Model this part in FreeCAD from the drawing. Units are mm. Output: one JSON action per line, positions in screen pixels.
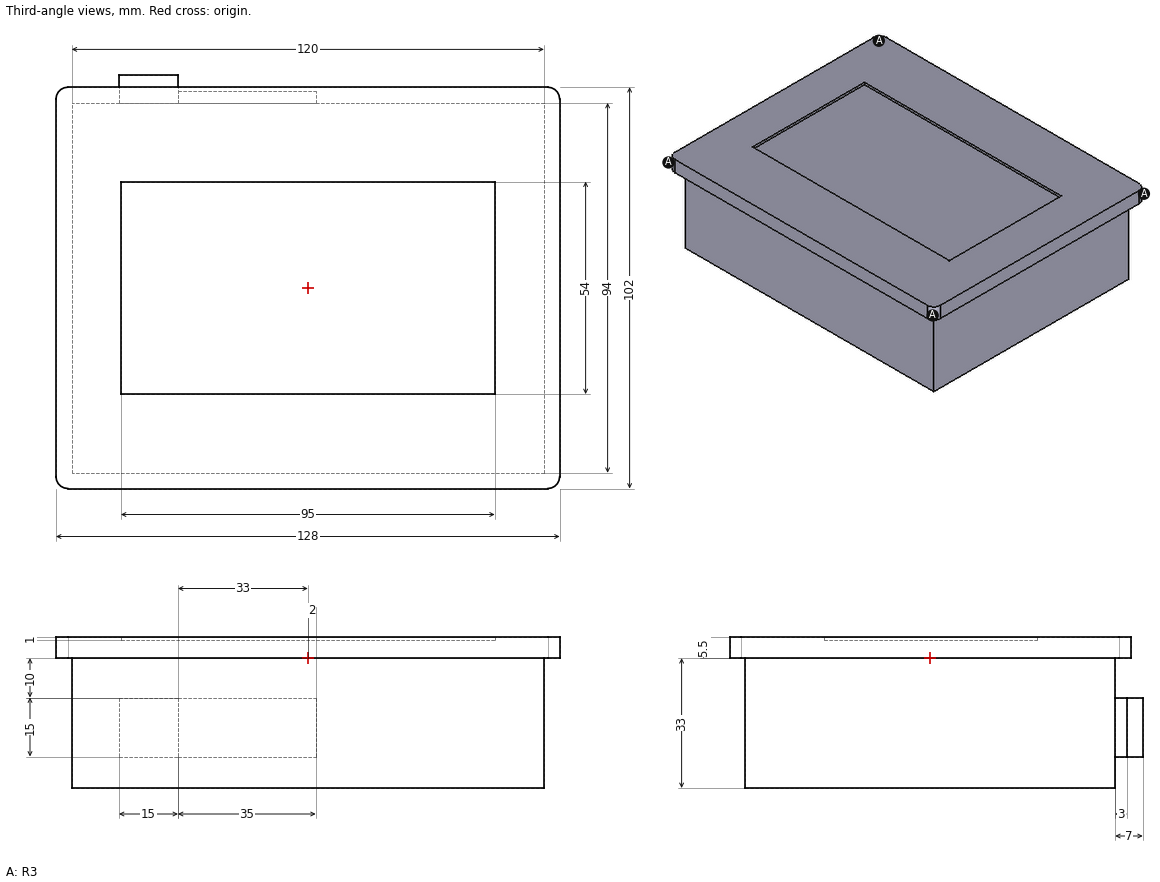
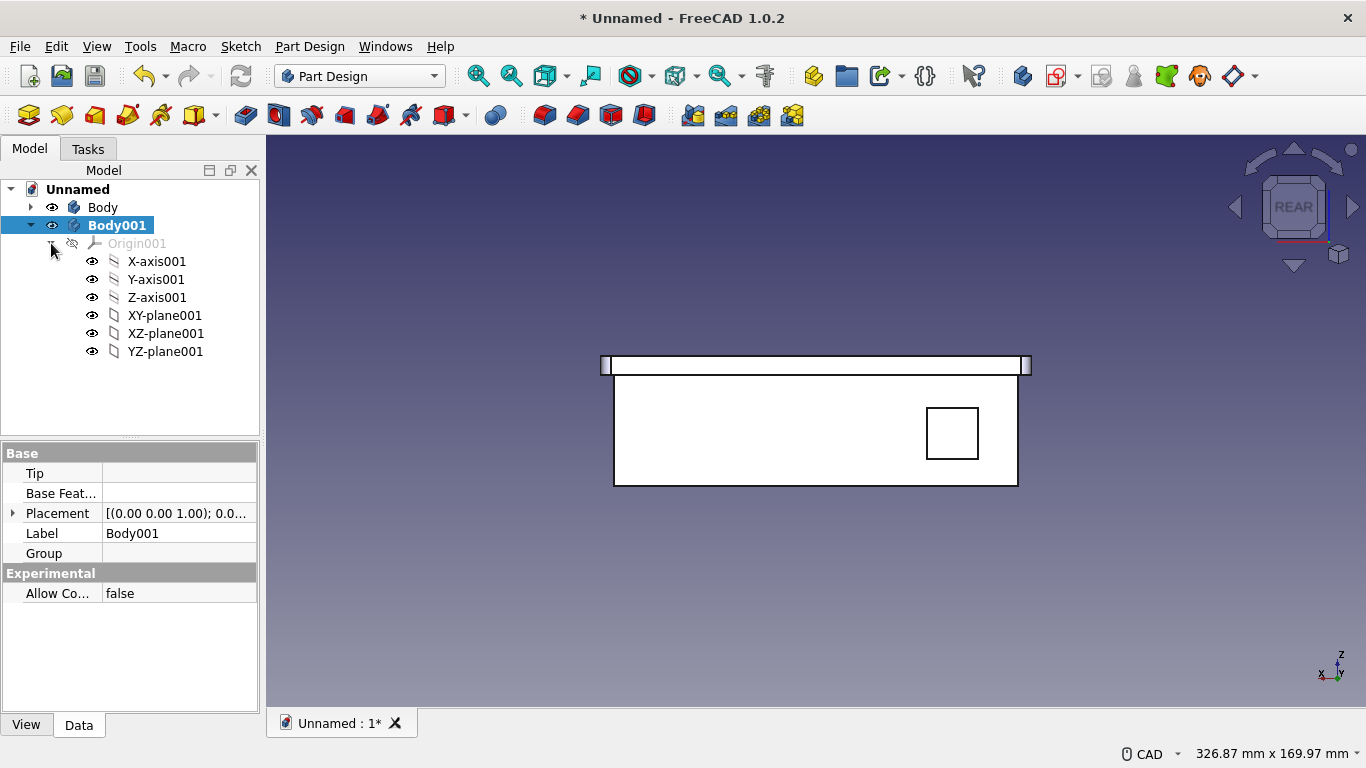
{"action": "left_click", "coordinate": [137, 333]}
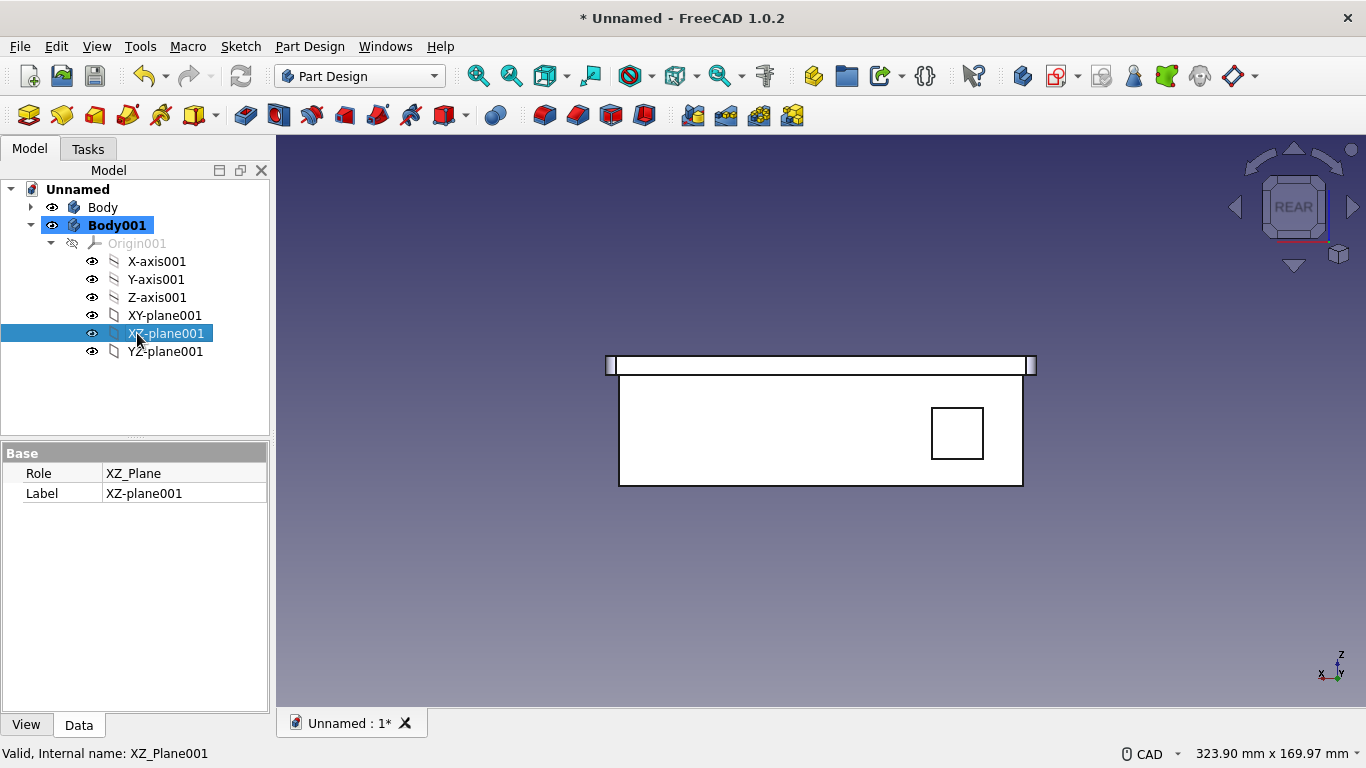
{"action": "left_click", "coordinate": [1232, 76]}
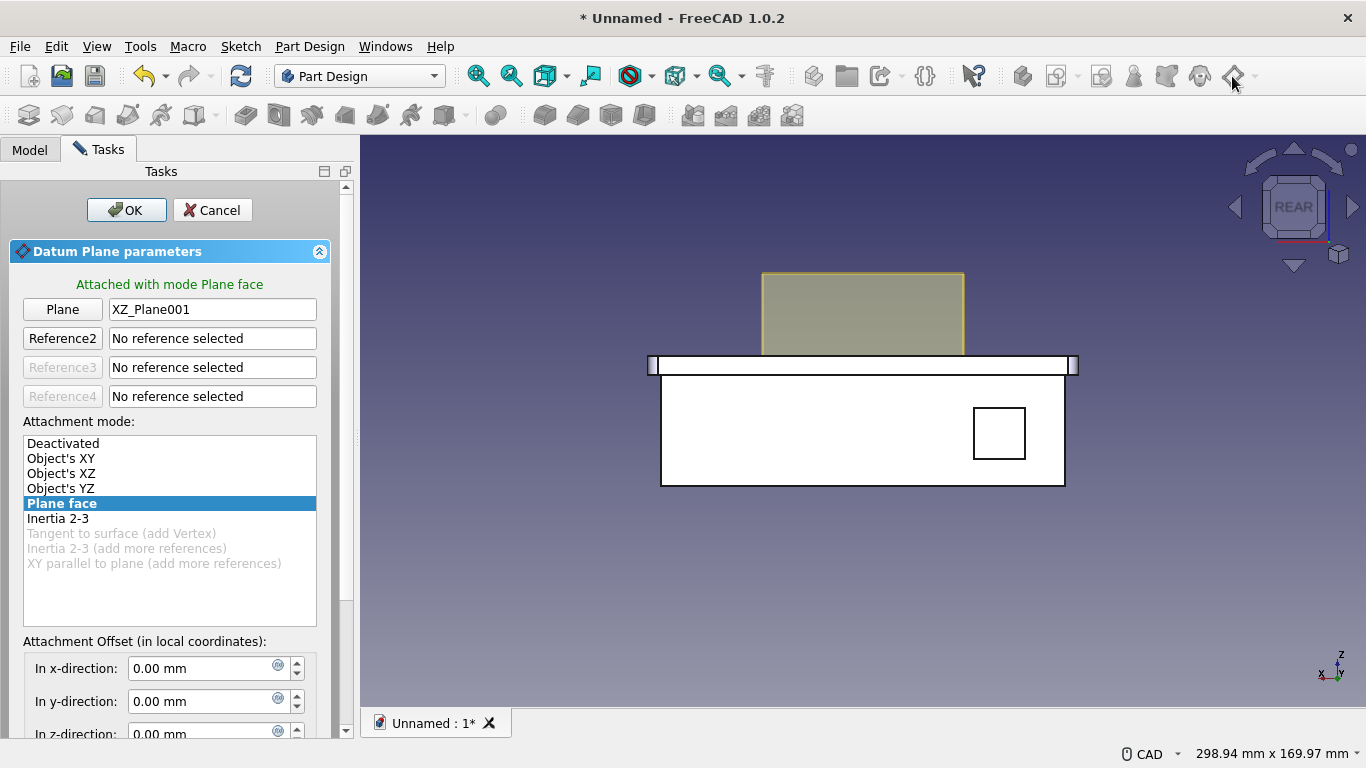
{"action": "scroll", "coordinate": [346, 460], "scroll_direction": "down", "scroll_amount": 2}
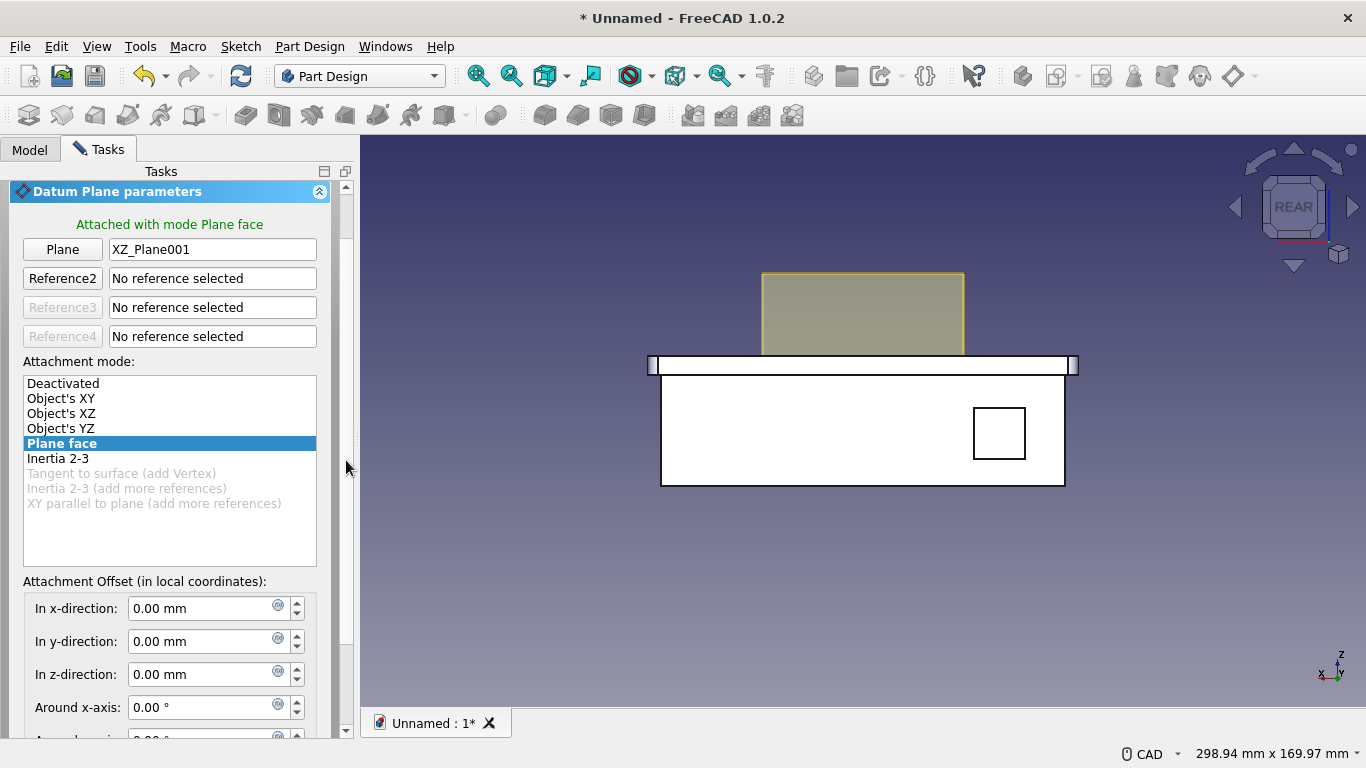
{"action": "triple_click", "coordinate": [210, 614]}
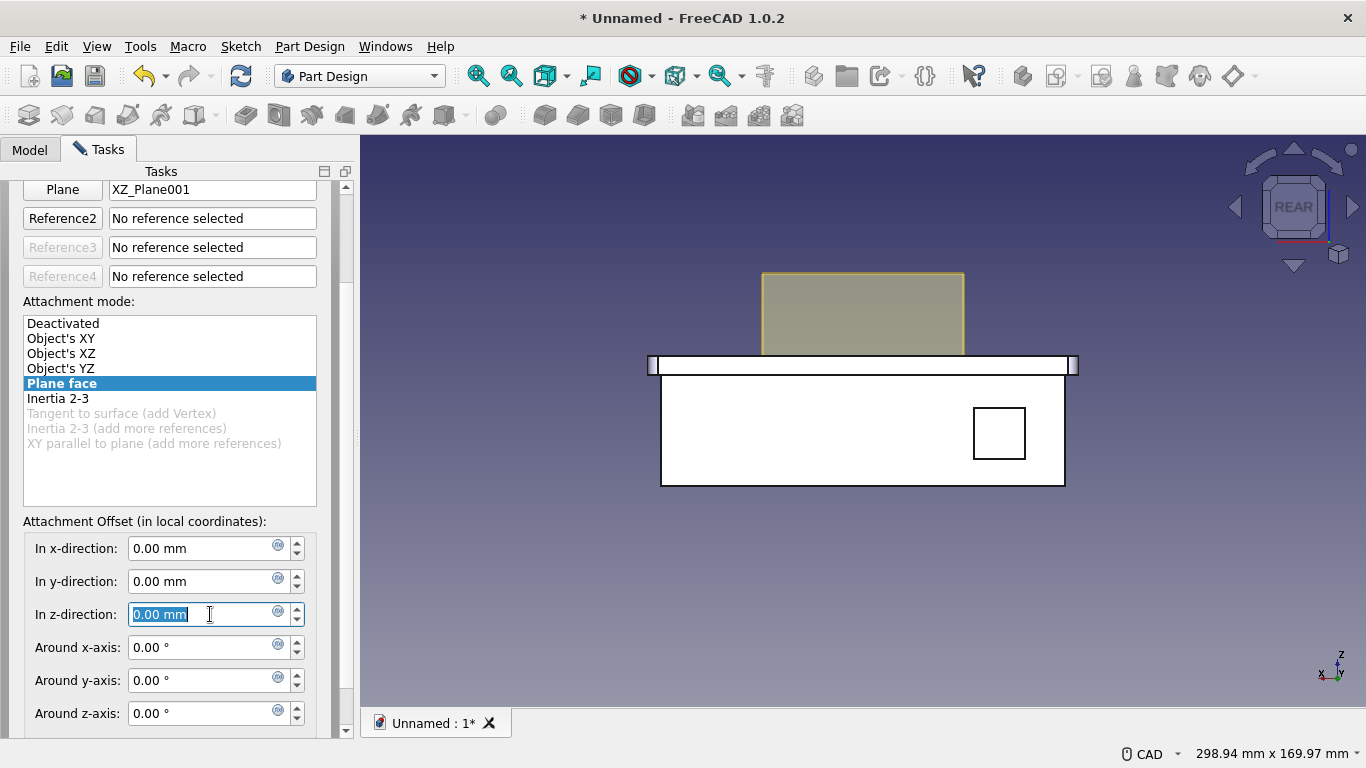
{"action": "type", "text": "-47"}
{"action": "key", "text": "Tab"}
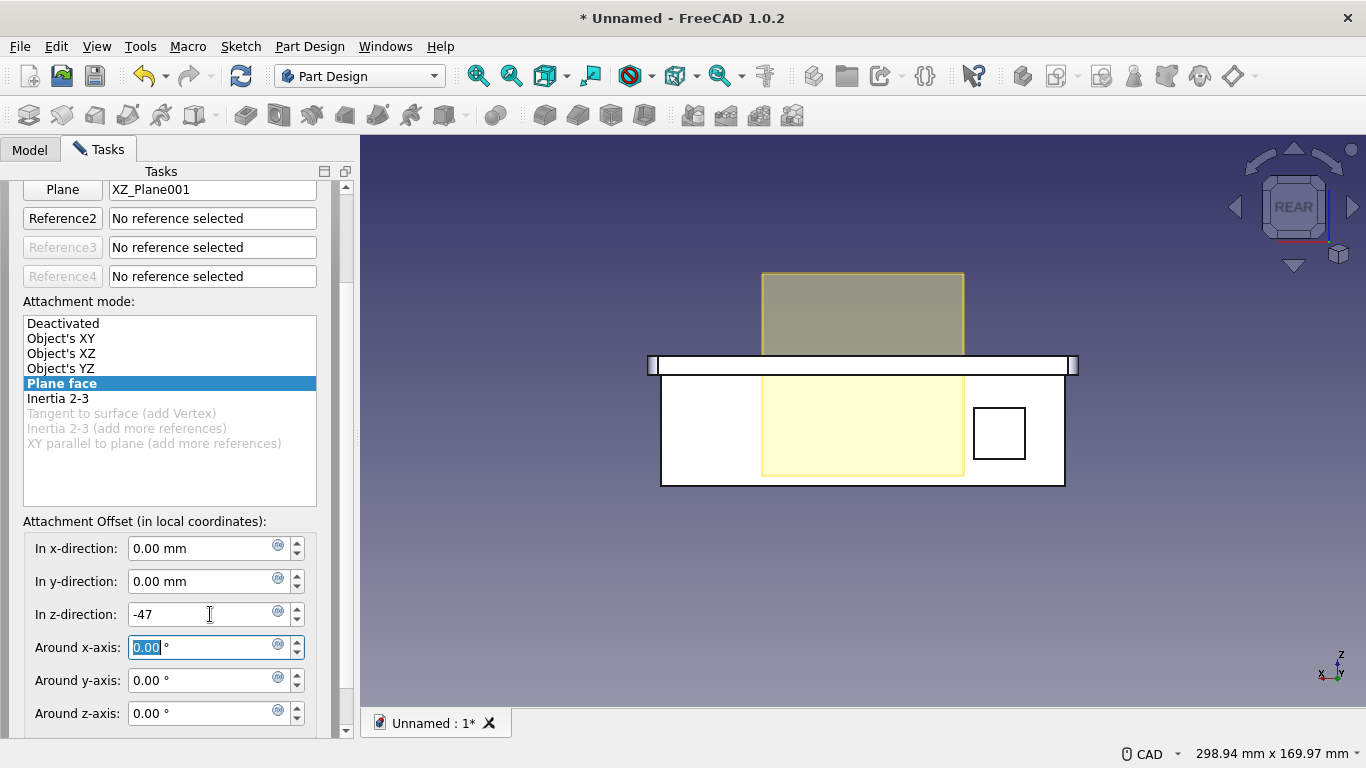
{"action": "scroll", "coordinate": [346, 460], "scroll_direction": "up", "scroll_amount": 3}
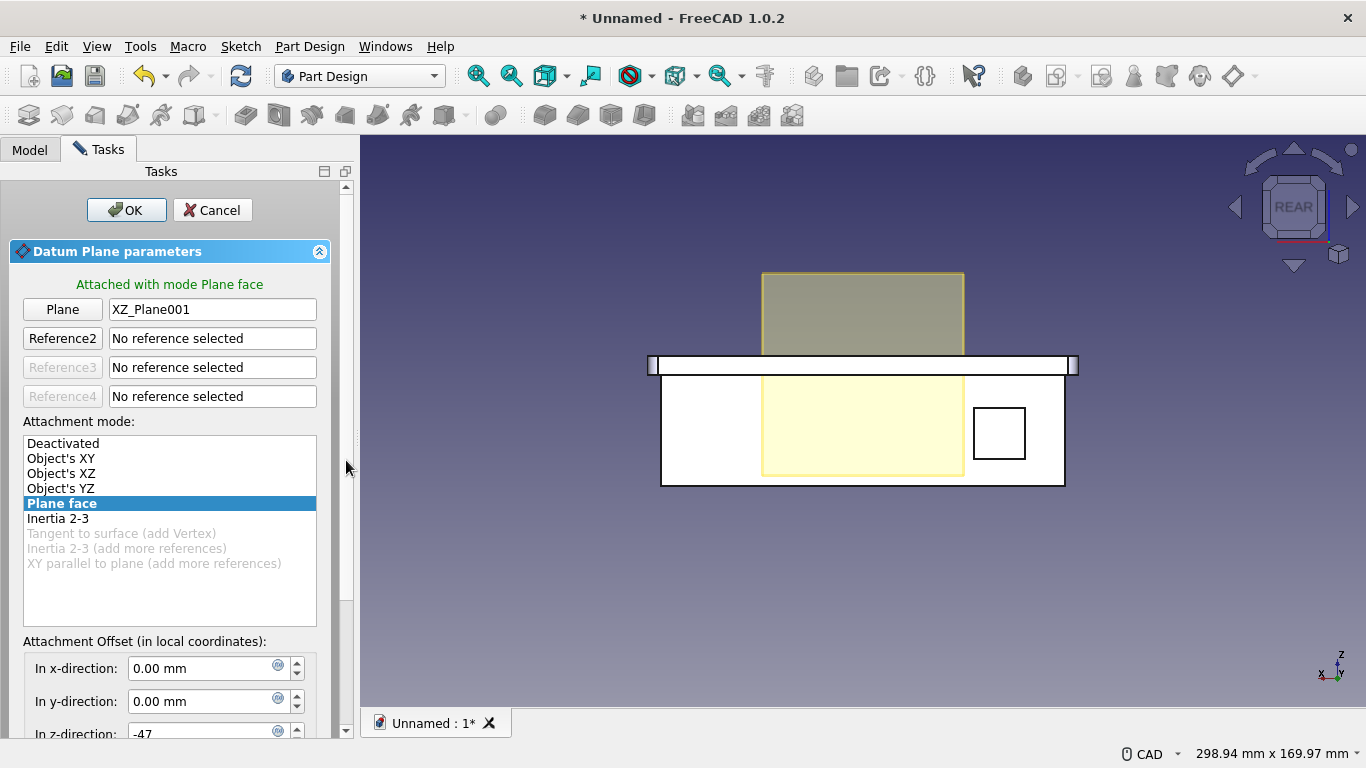
{"action": "left_click", "coordinate": [127, 210]}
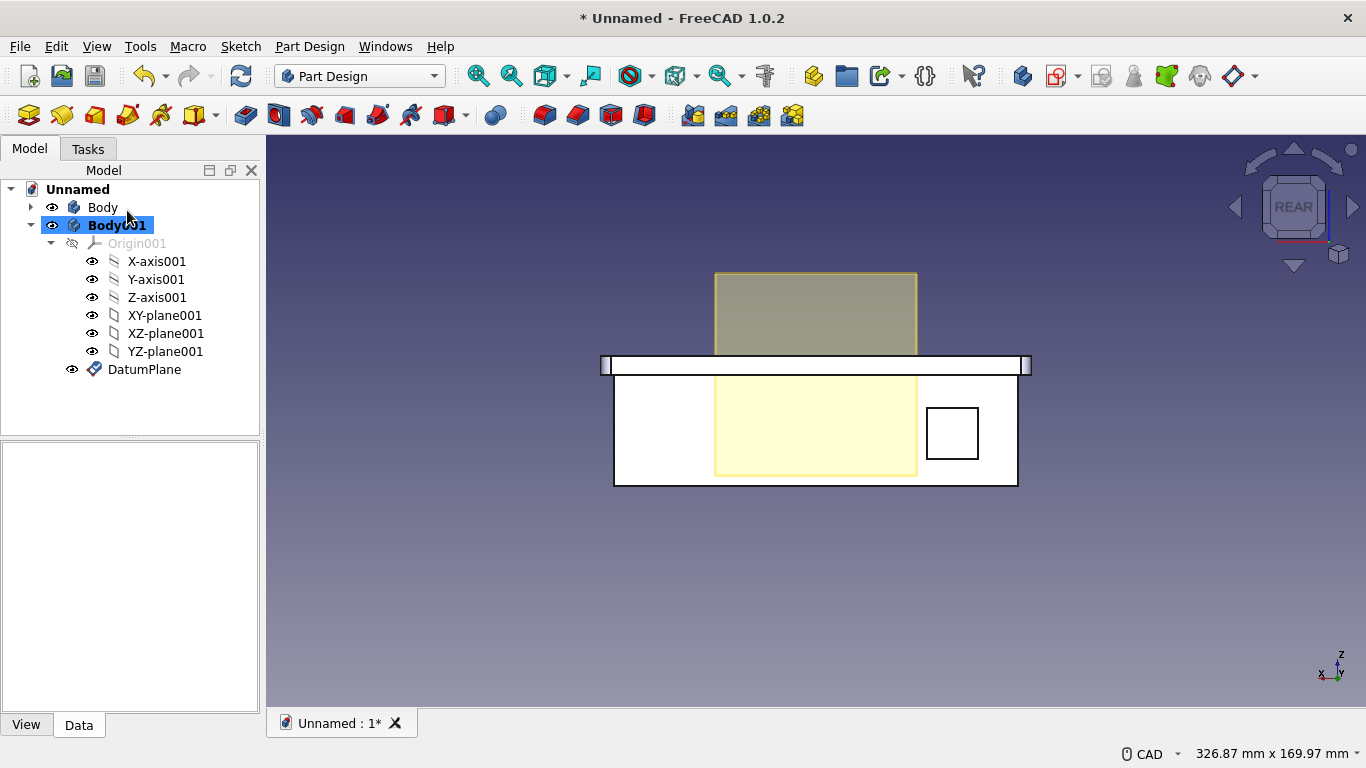
{"action": "left_click", "coordinate": [117, 369]}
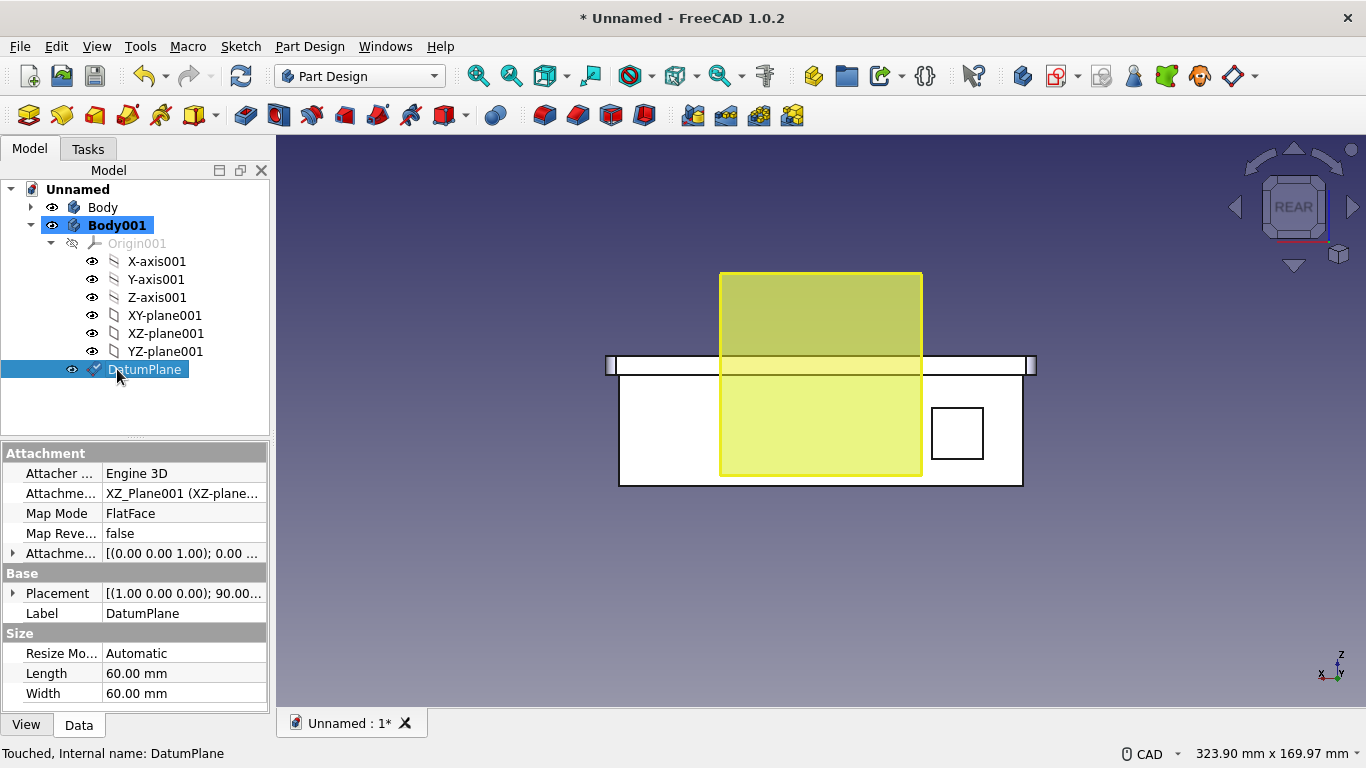
{"action": "left_click", "coordinate": [1056, 76]}